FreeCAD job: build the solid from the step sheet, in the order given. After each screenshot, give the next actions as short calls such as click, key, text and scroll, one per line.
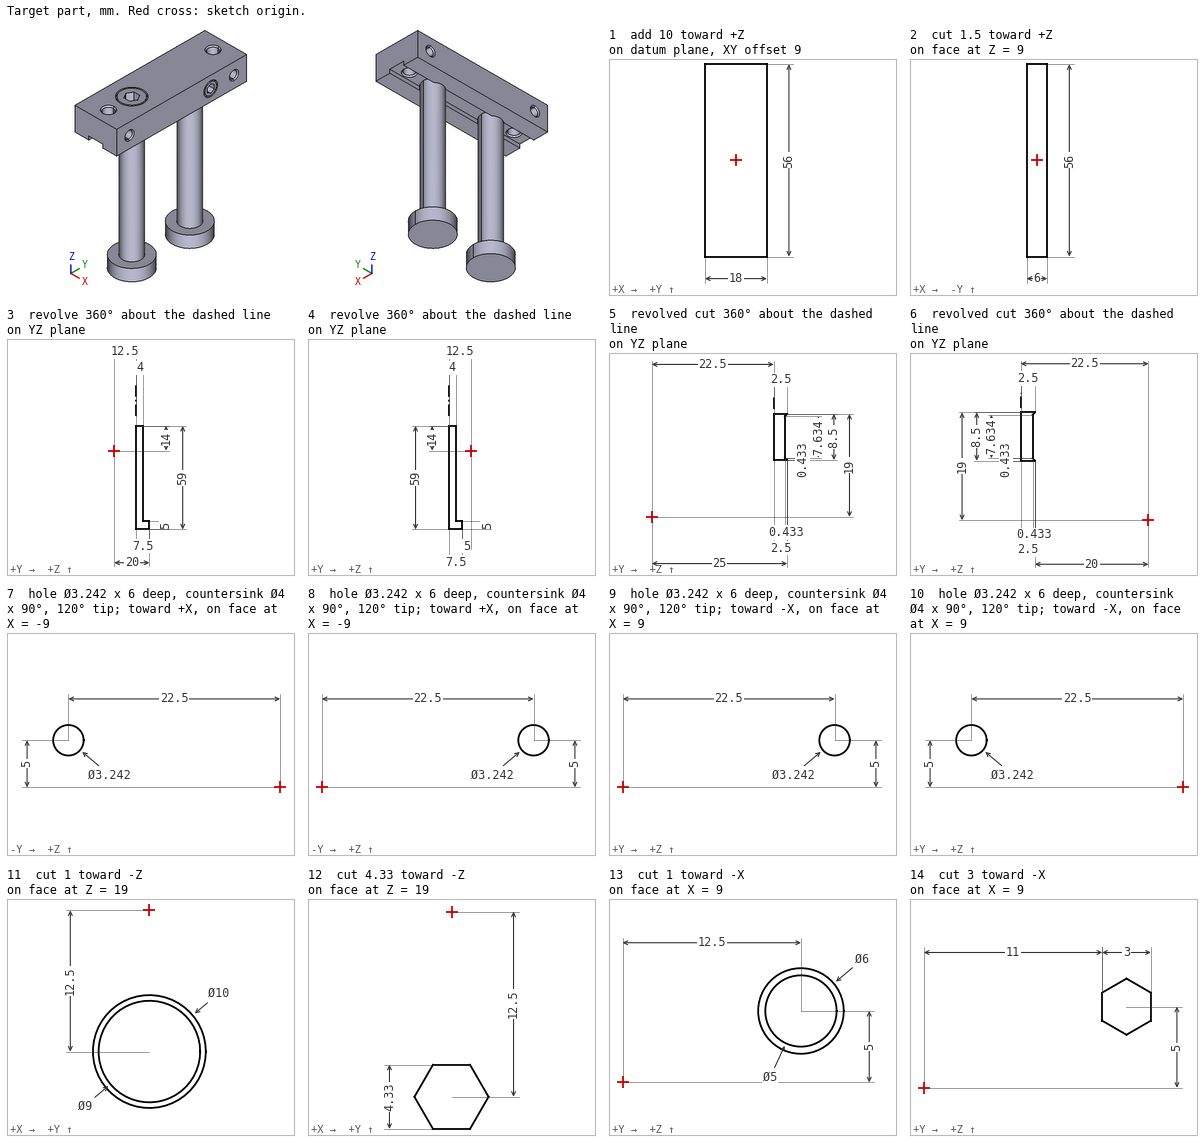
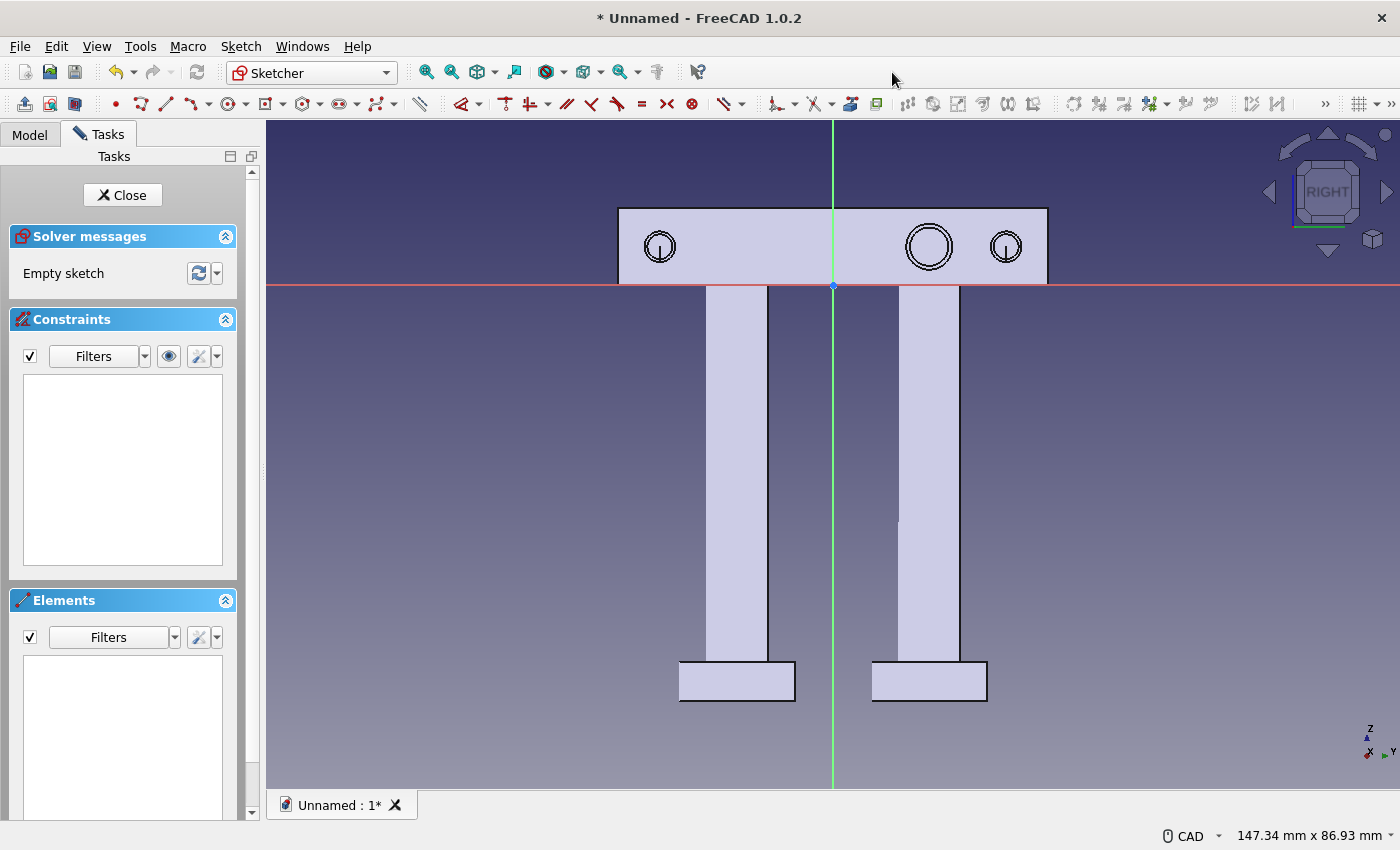
scroll(940, 233, up, 14)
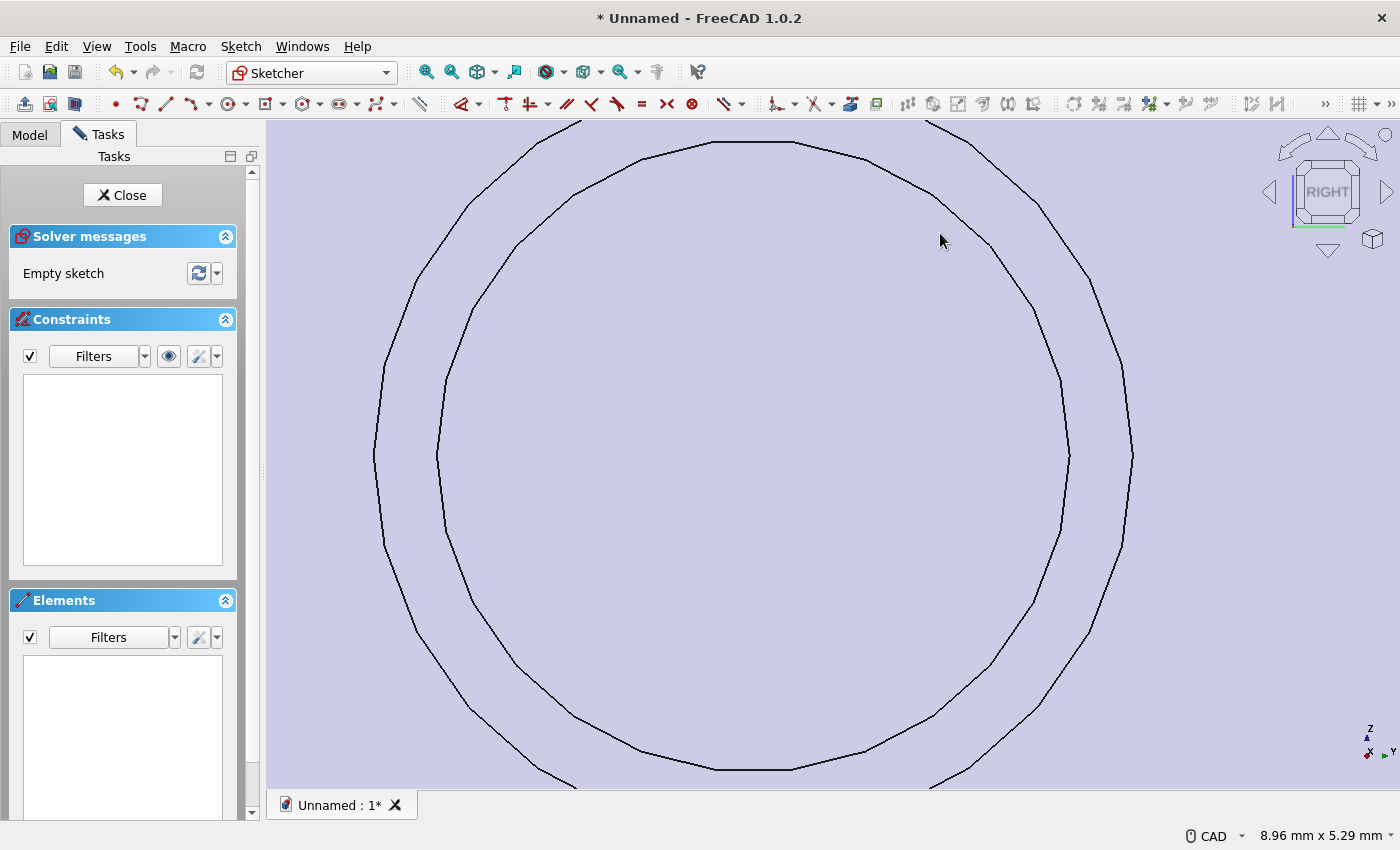
click(302, 104)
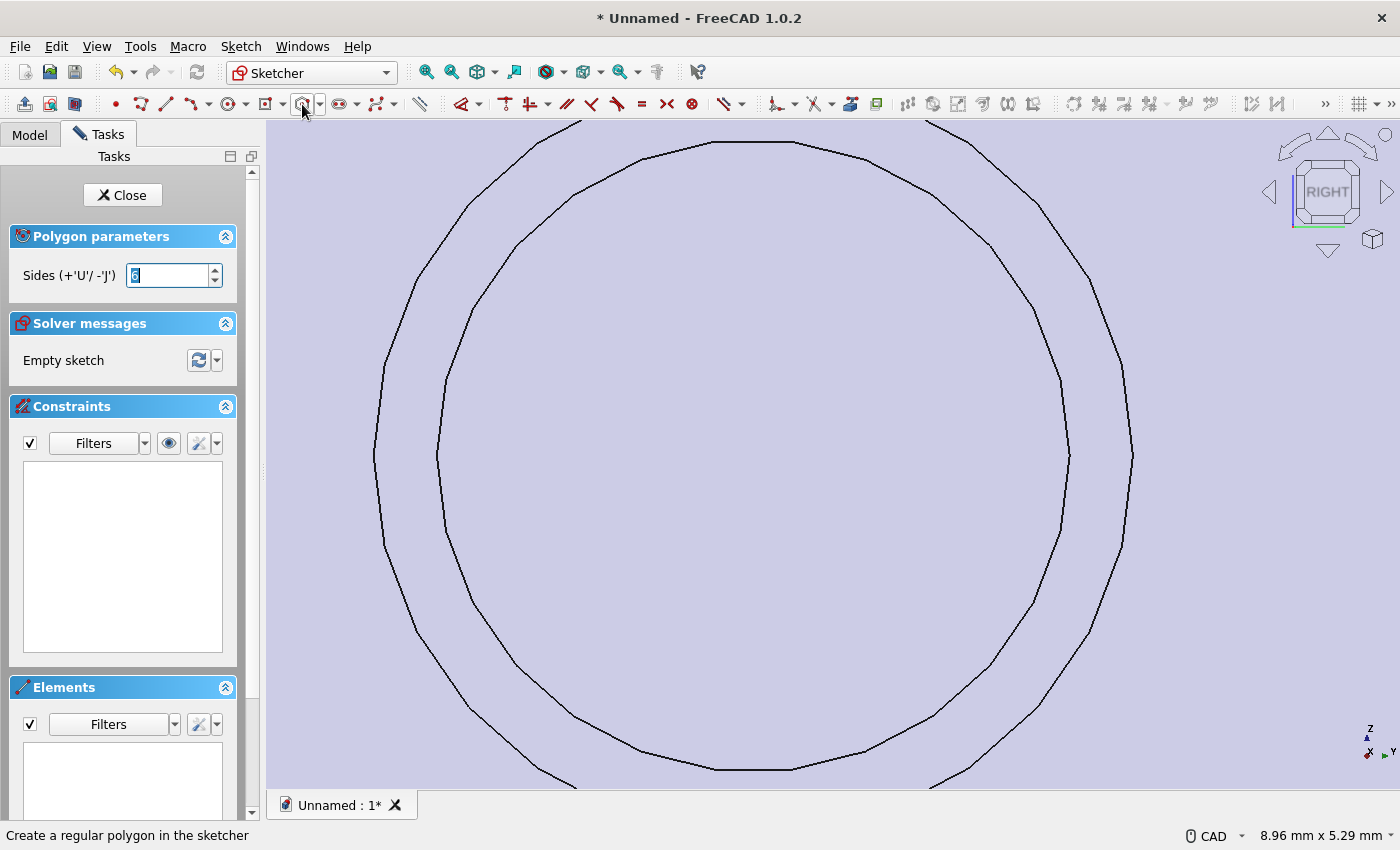
click(753, 456)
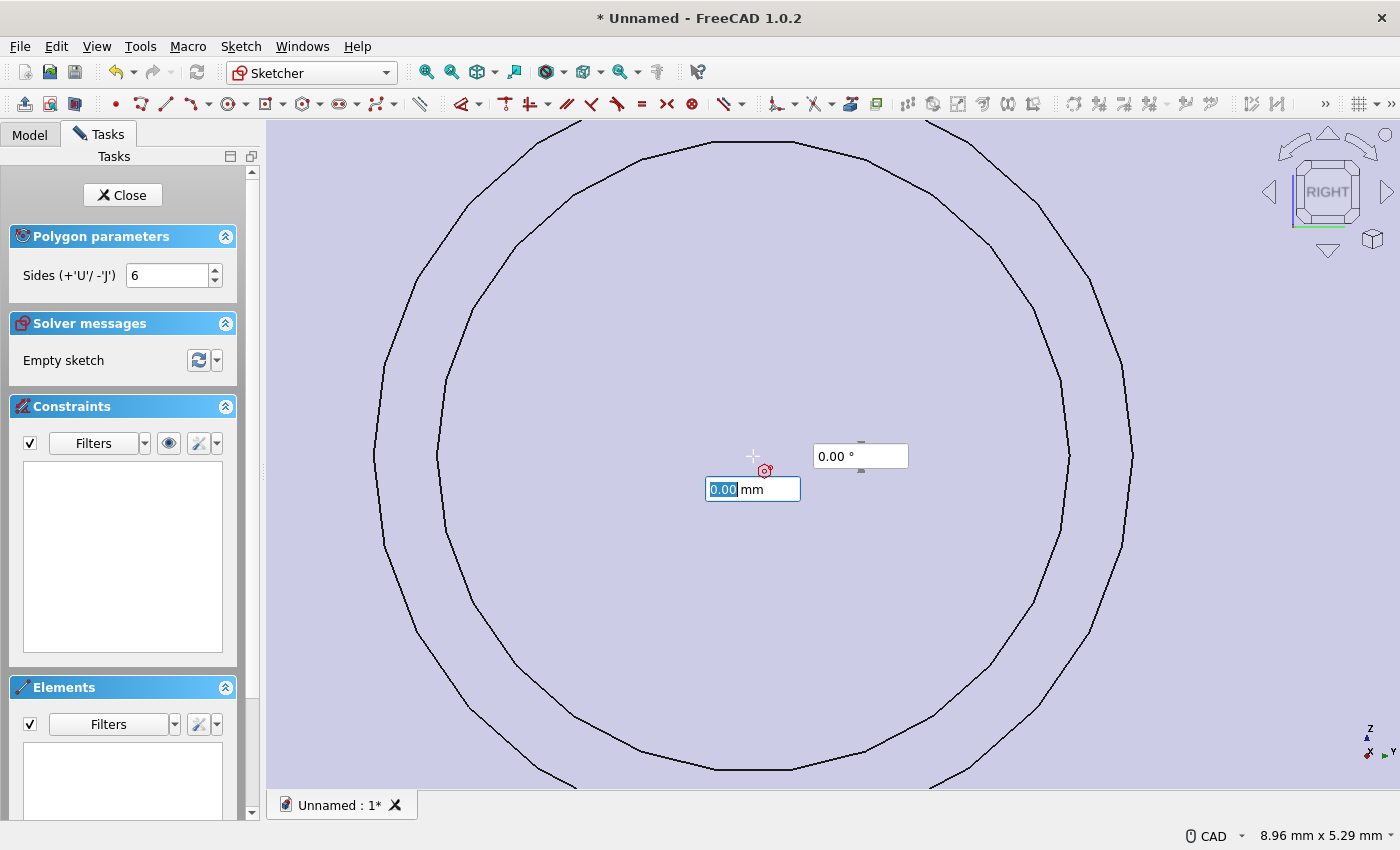
click(753, 236)
right_click(753, 236)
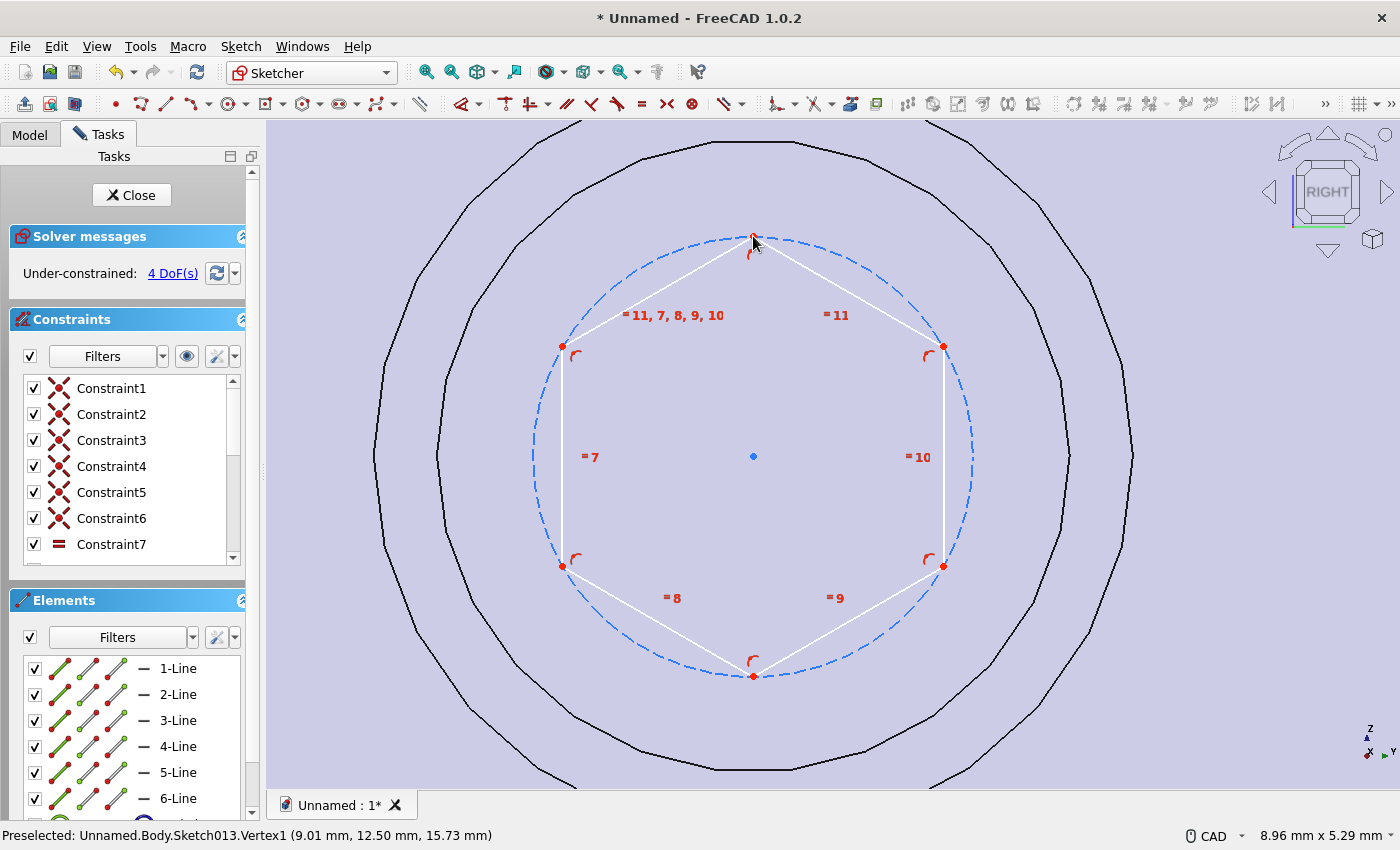
click(562, 413)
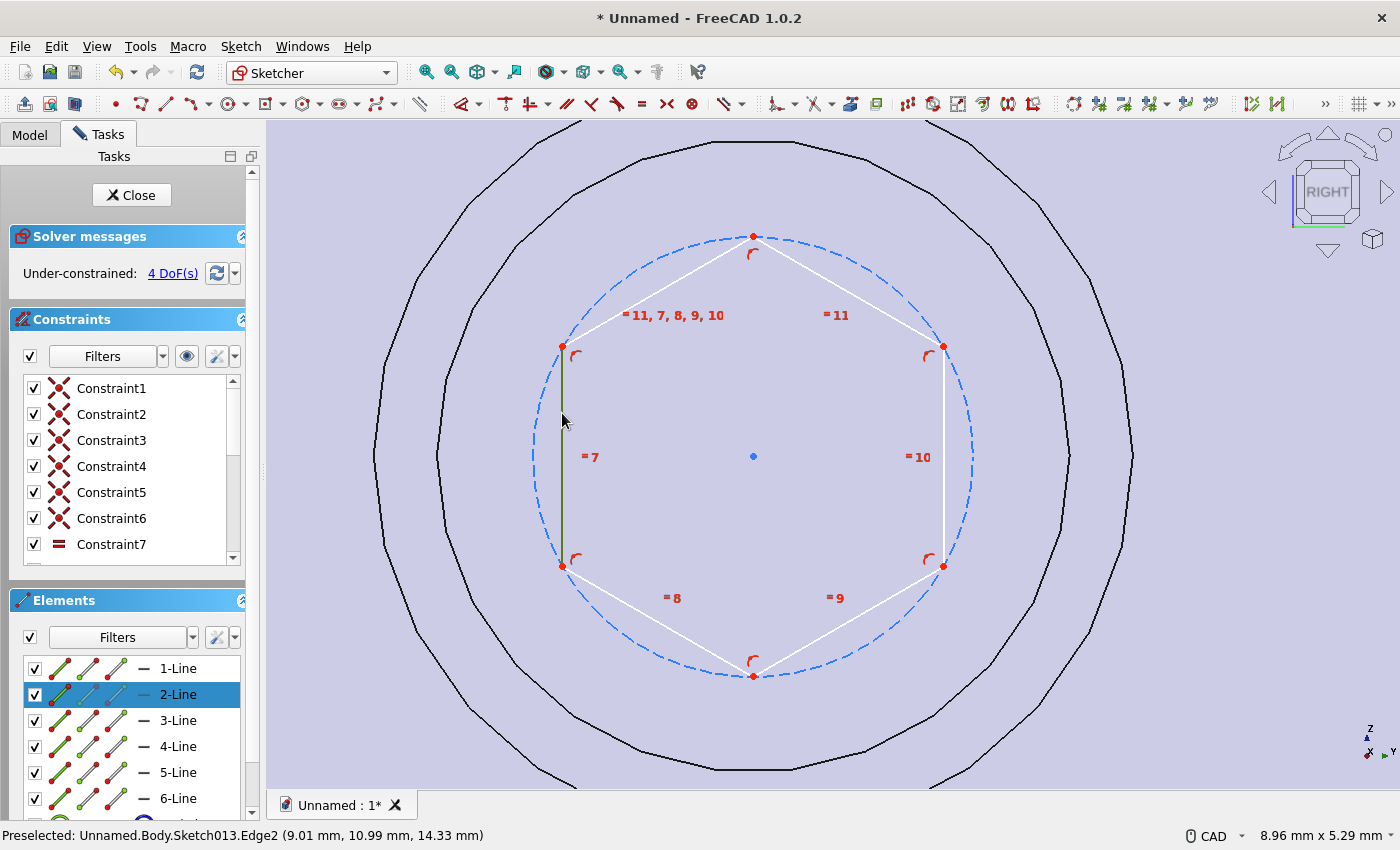
click(548, 104)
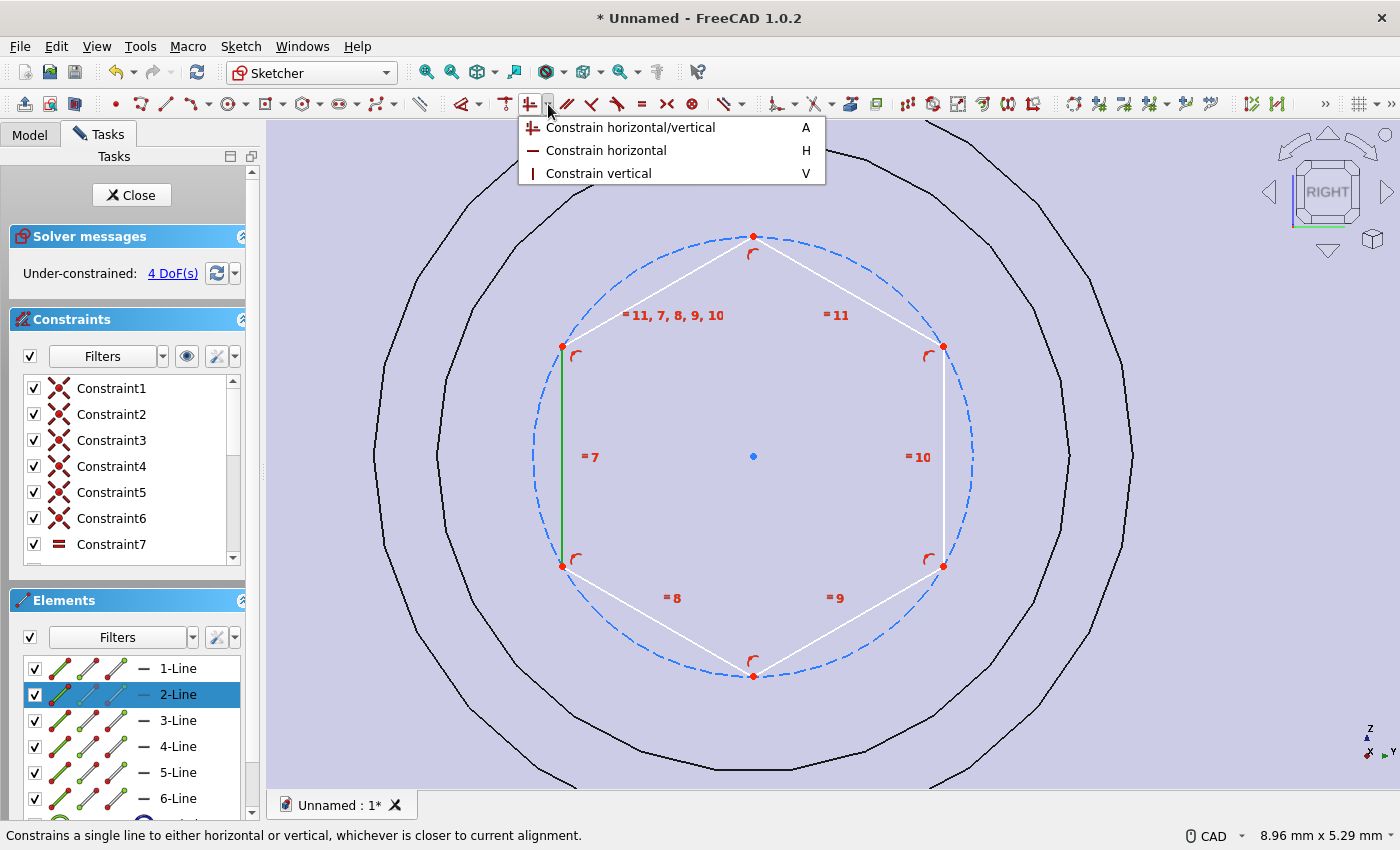
click(672, 174)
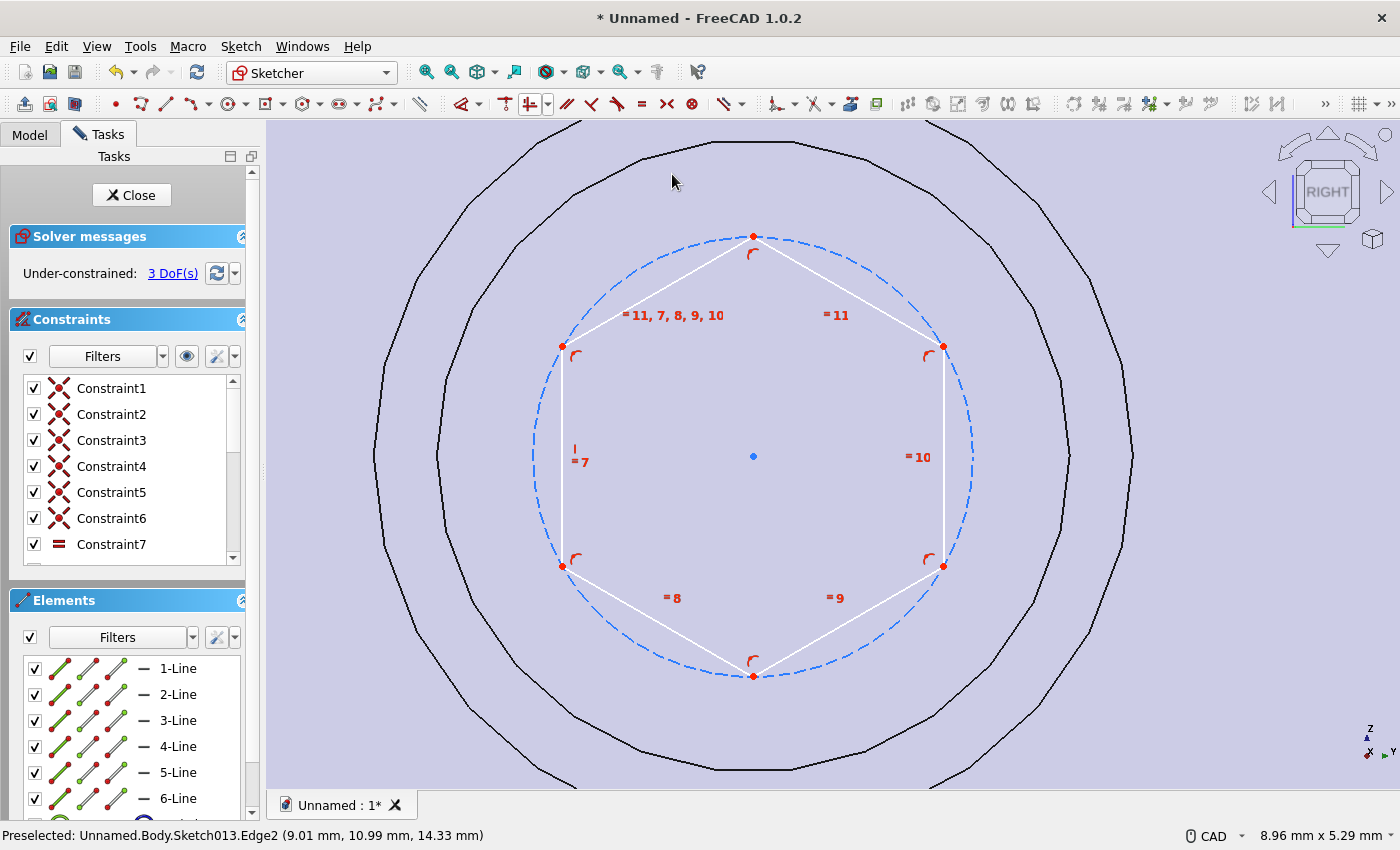
click(460, 104)